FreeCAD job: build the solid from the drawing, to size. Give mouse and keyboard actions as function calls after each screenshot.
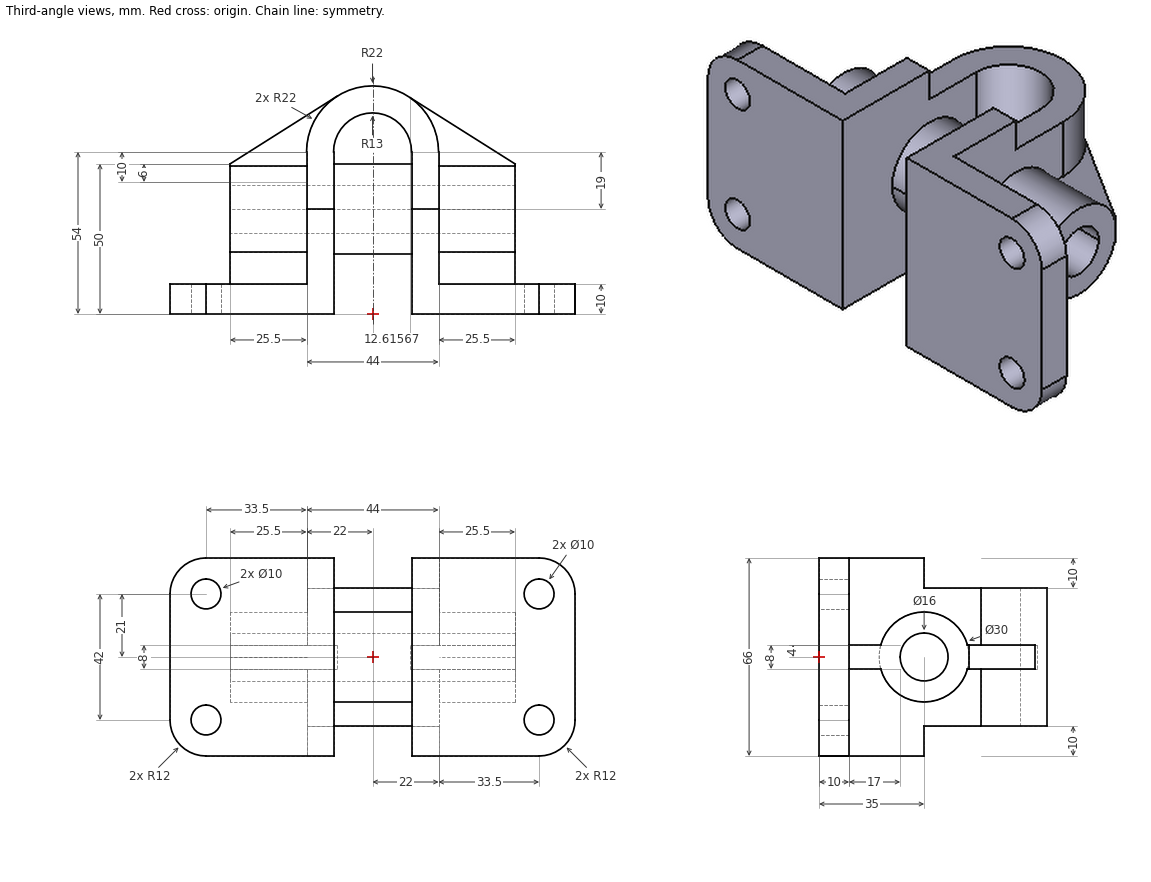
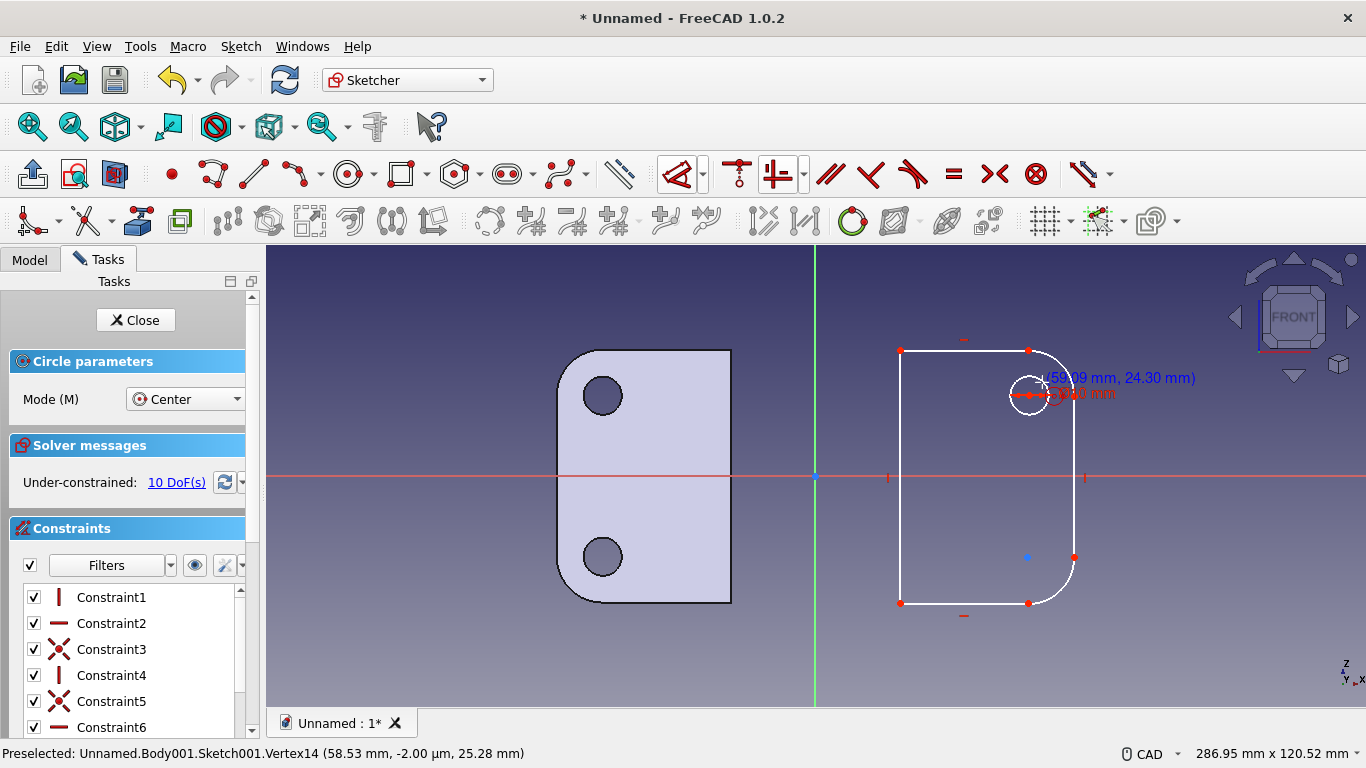
click(1028, 557)
move(1042, 543)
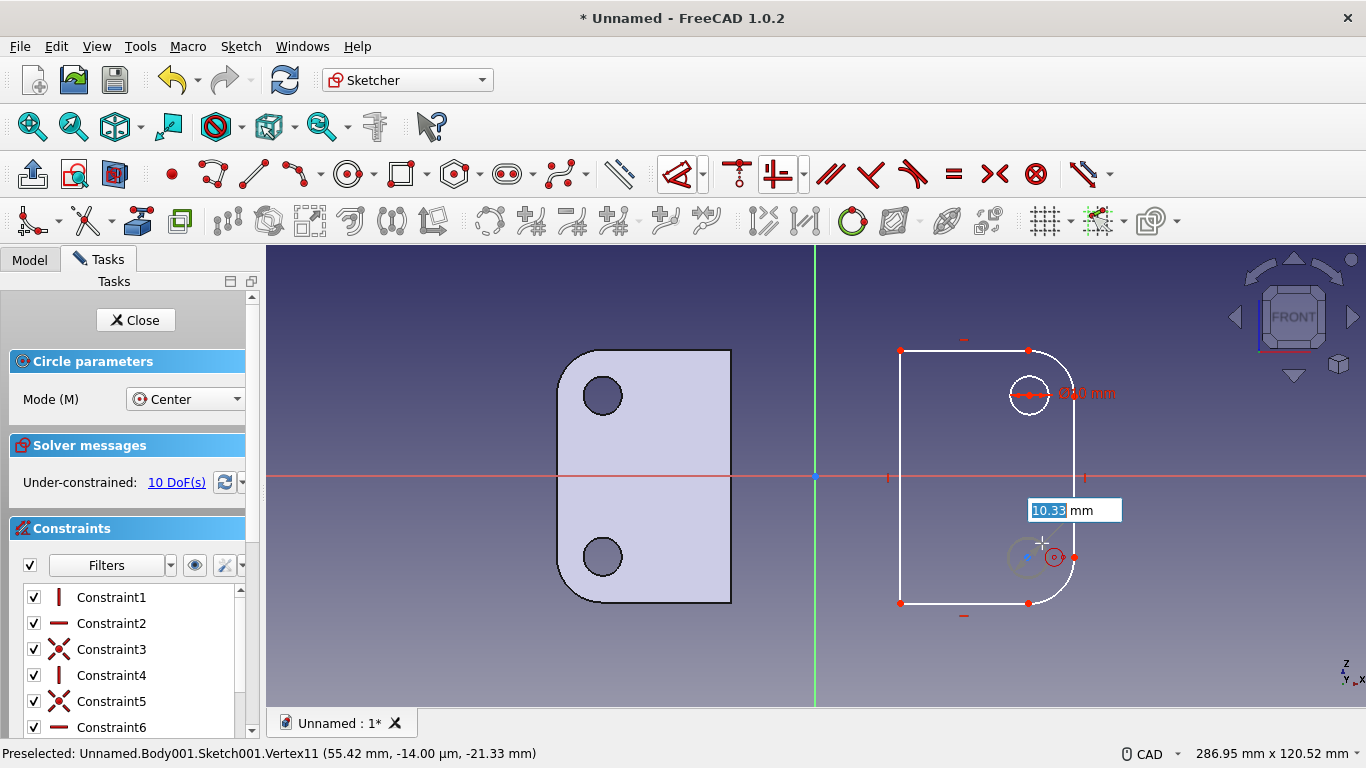
text(10)
key(Return)
key(Escape)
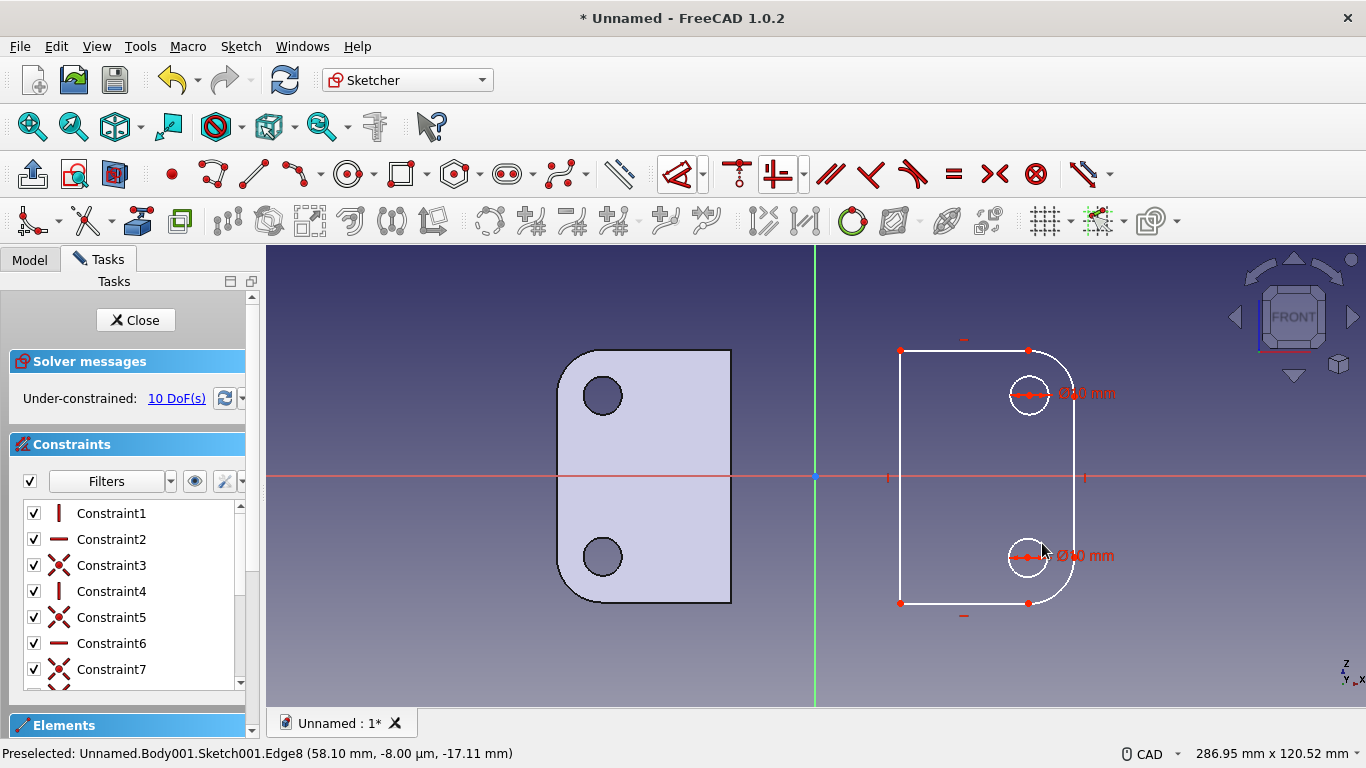
click(1074, 445)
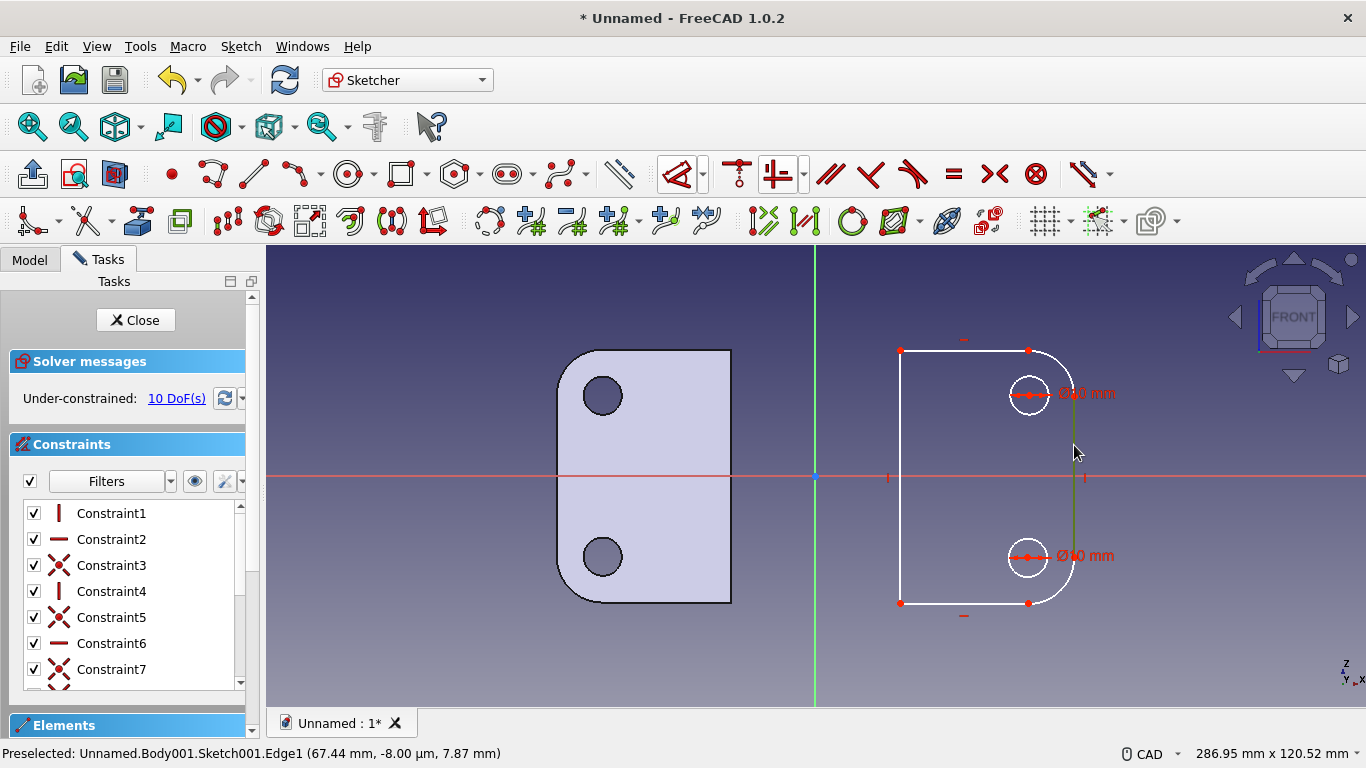
click(1049, 599)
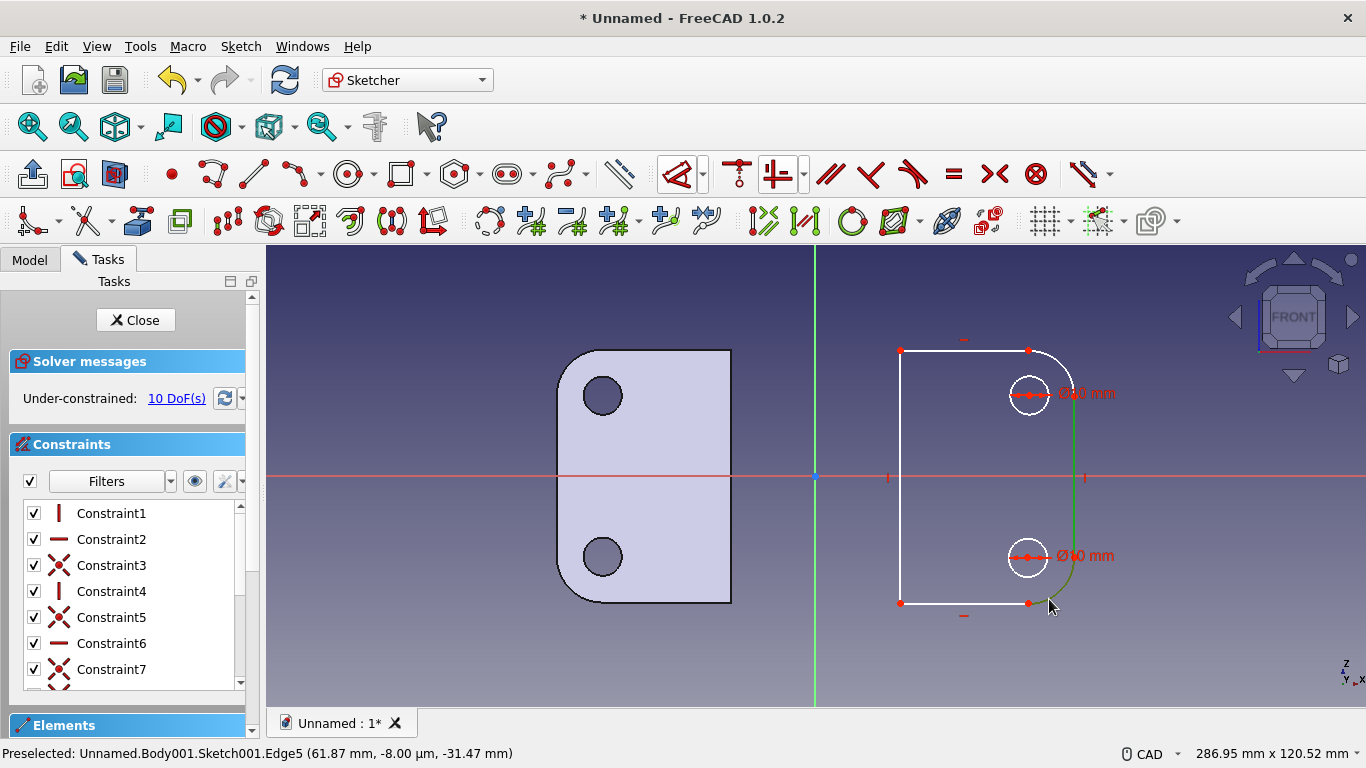
click(913, 174)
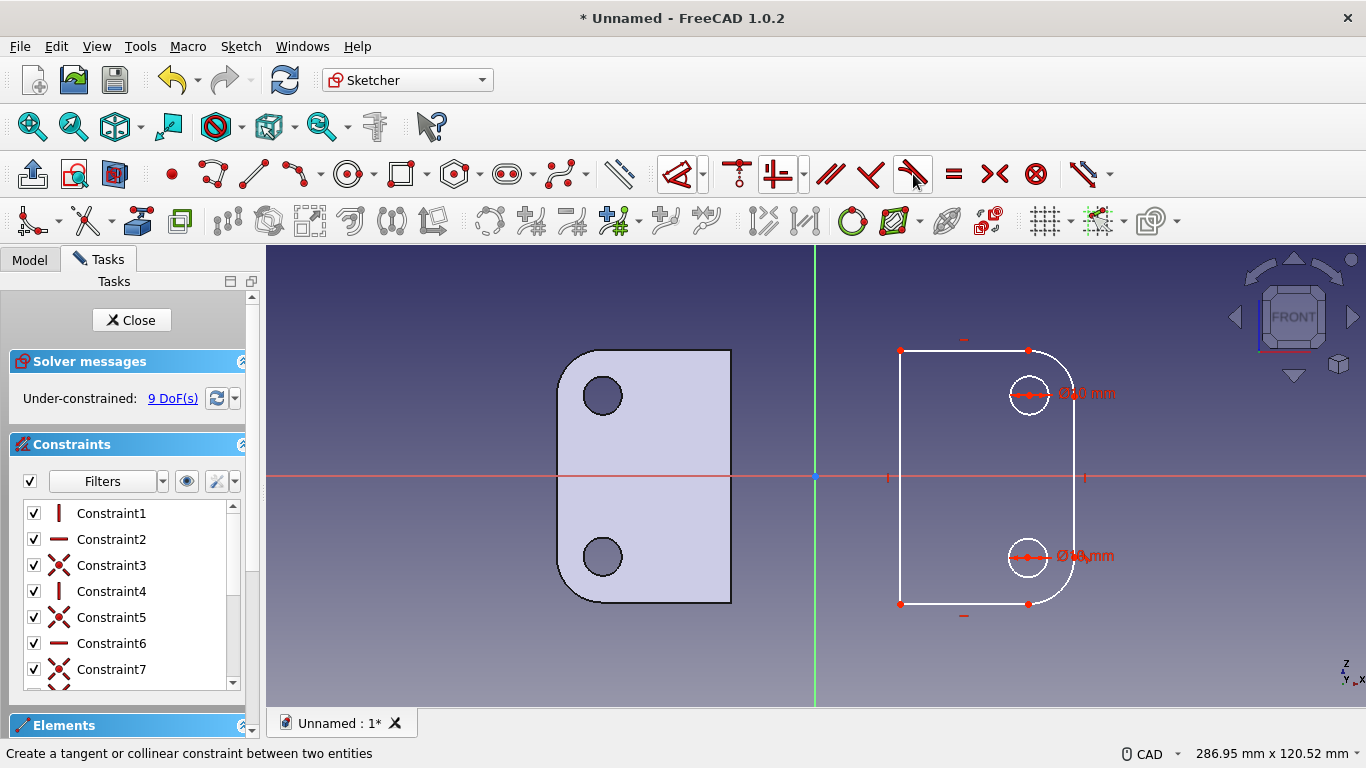
click(1074, 445)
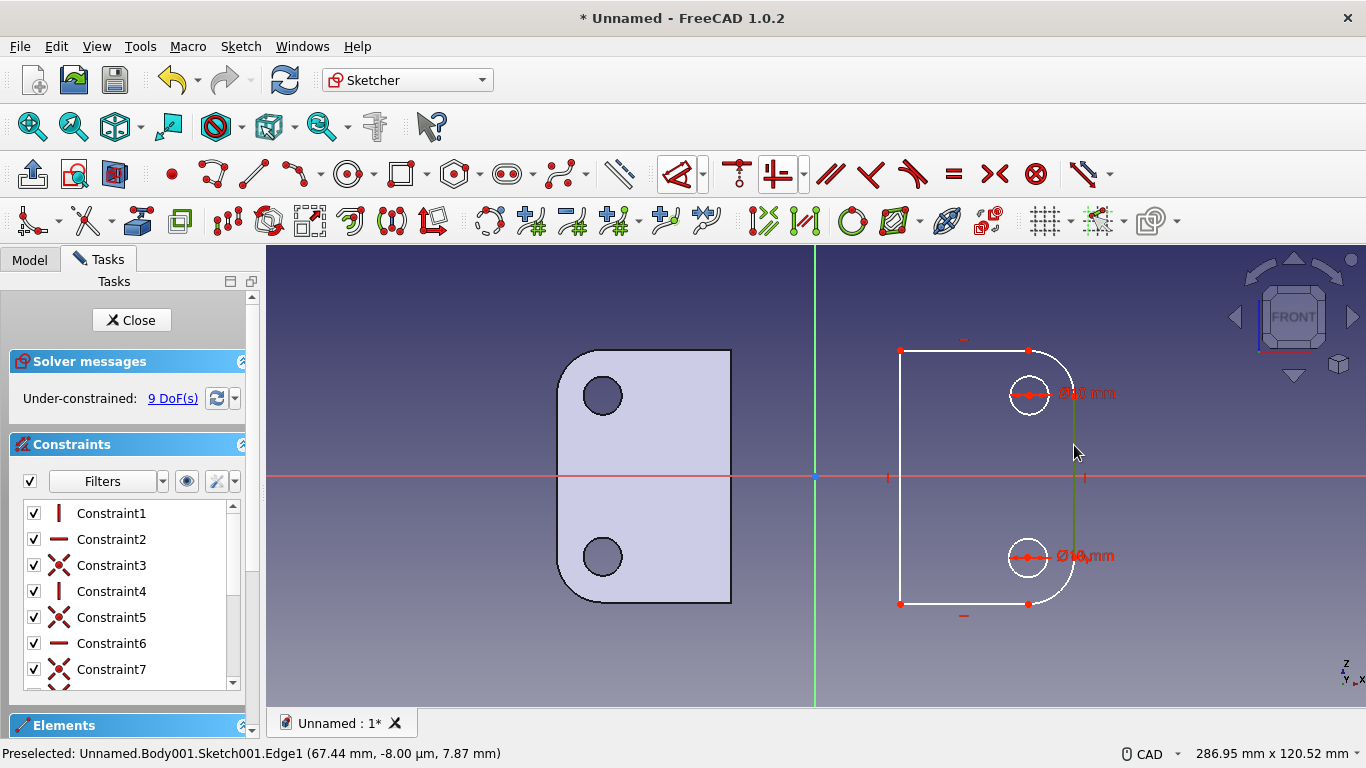
click(1069, 376)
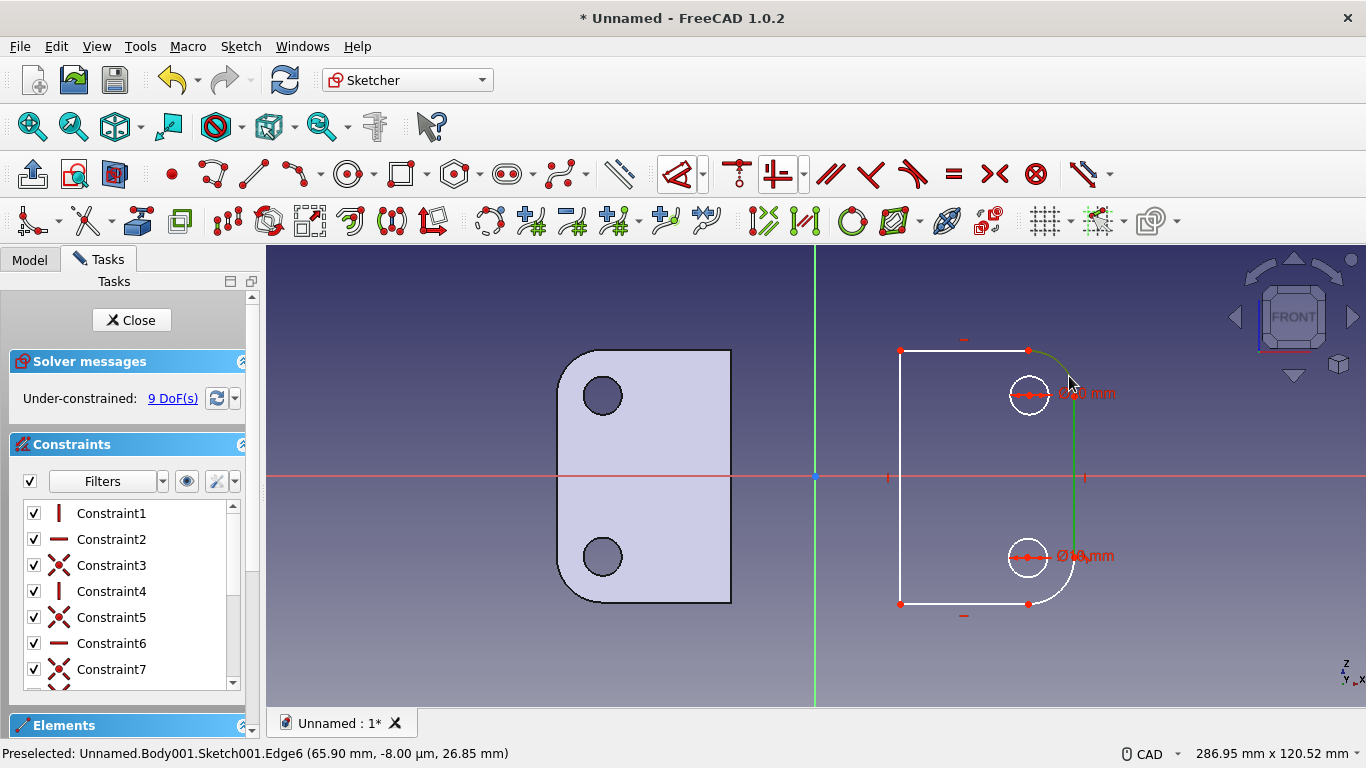
click(913, 174)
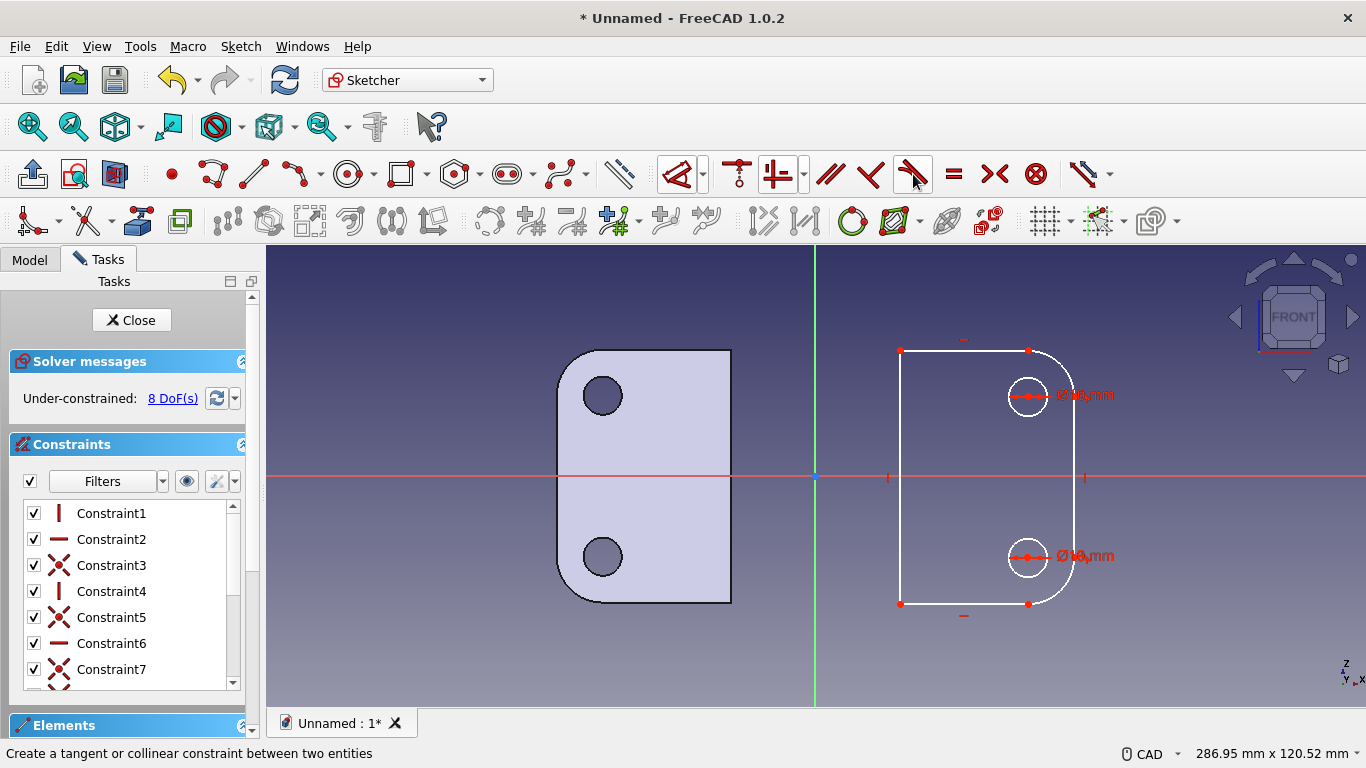
click(990, 604)